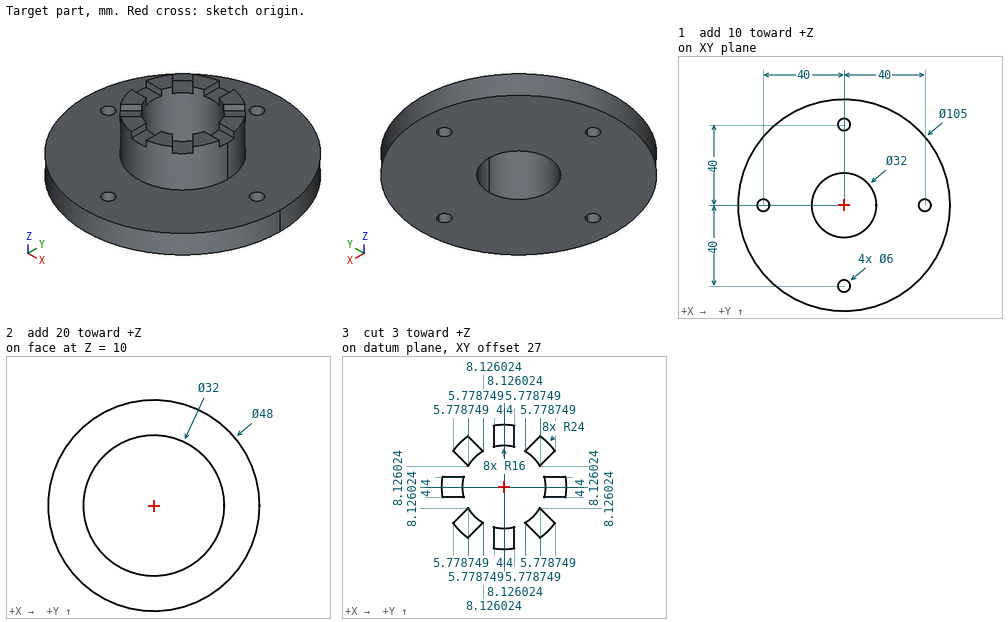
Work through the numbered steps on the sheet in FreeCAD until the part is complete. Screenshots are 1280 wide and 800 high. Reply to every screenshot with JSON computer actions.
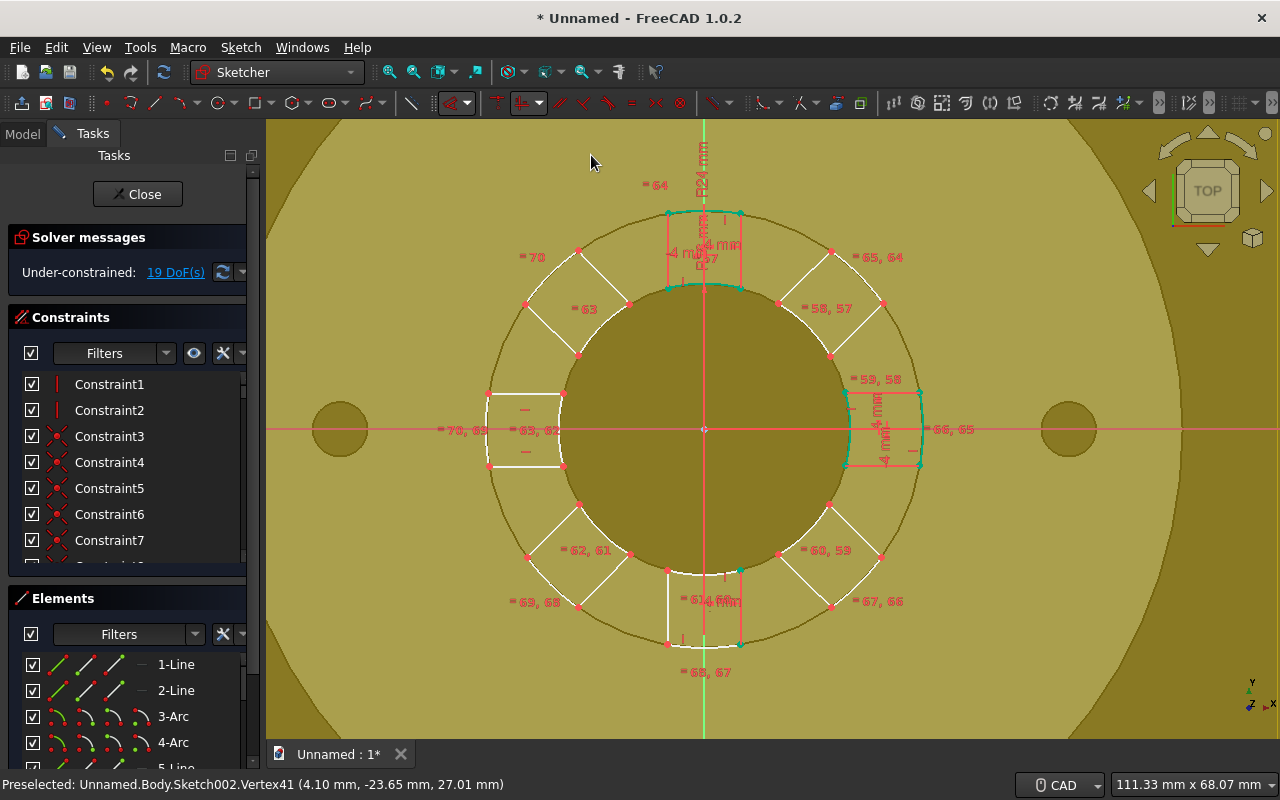
{"action": "left_click", "coordinate": [668, 570]}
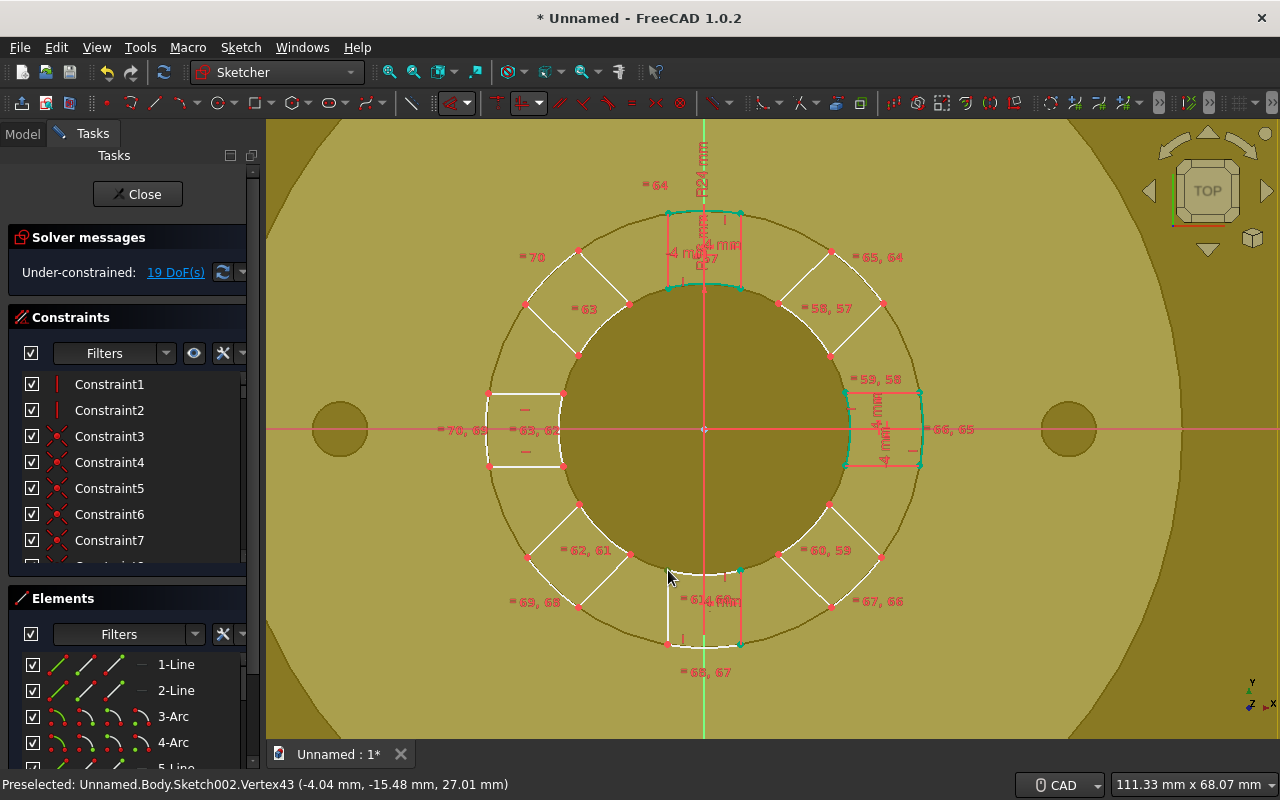
{"action": "left_click", "coordinate": [470, 104]}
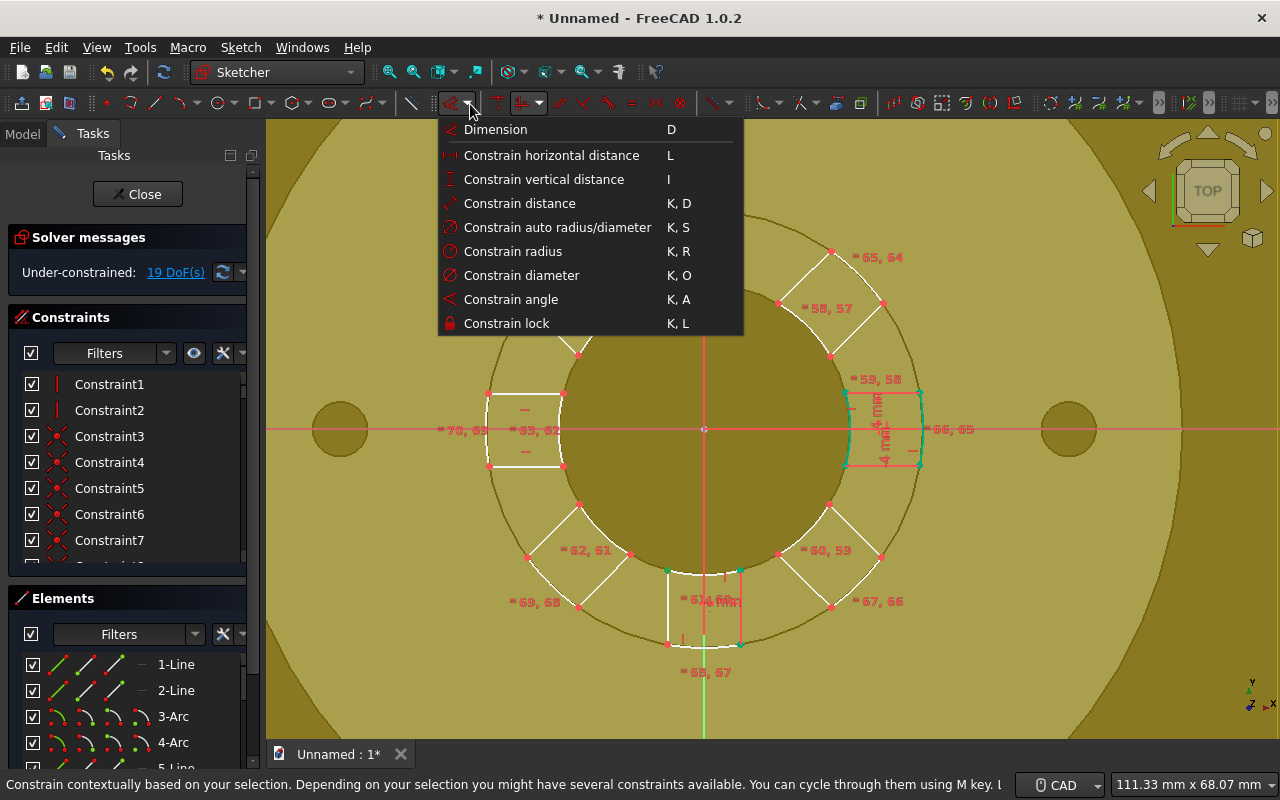
{"action": "left_click", "coordinate": [591, 155]}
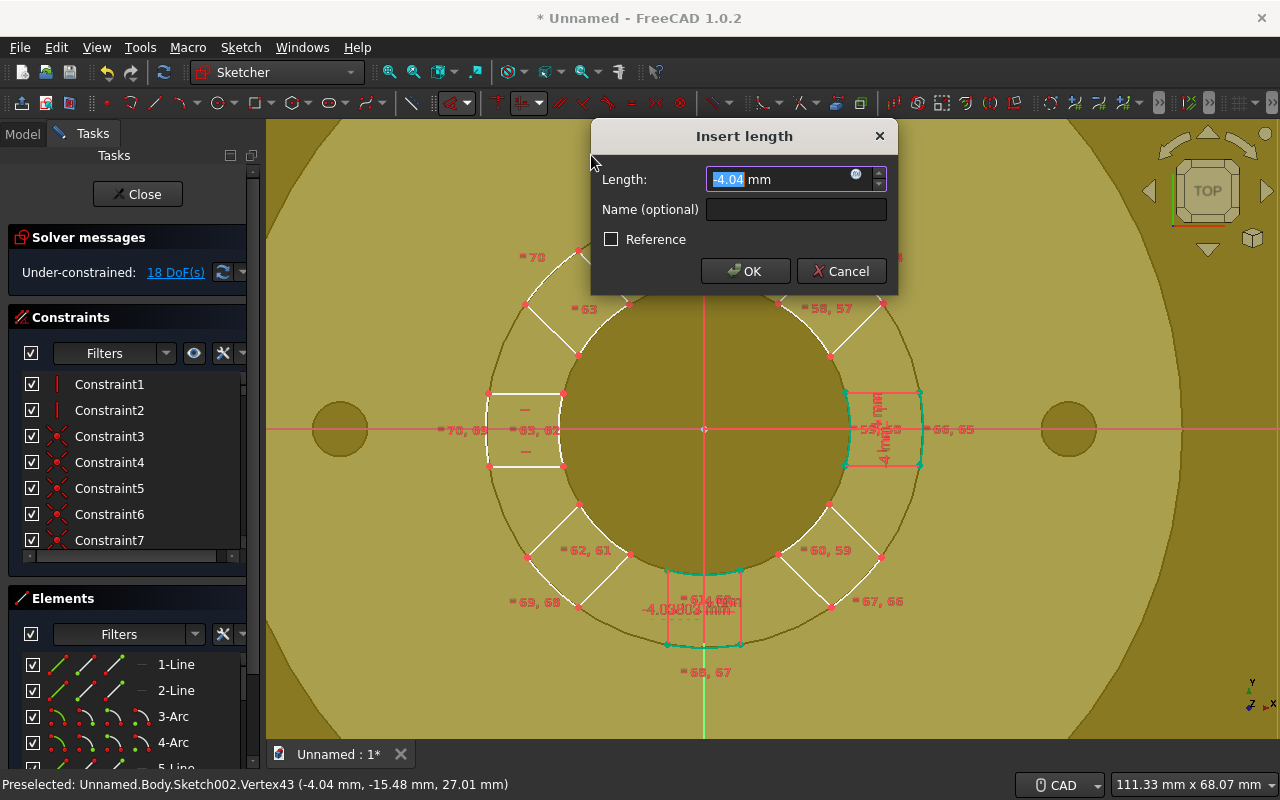
{"action": "type", "text": "-4"}
{"action": "key", "text": "Return"}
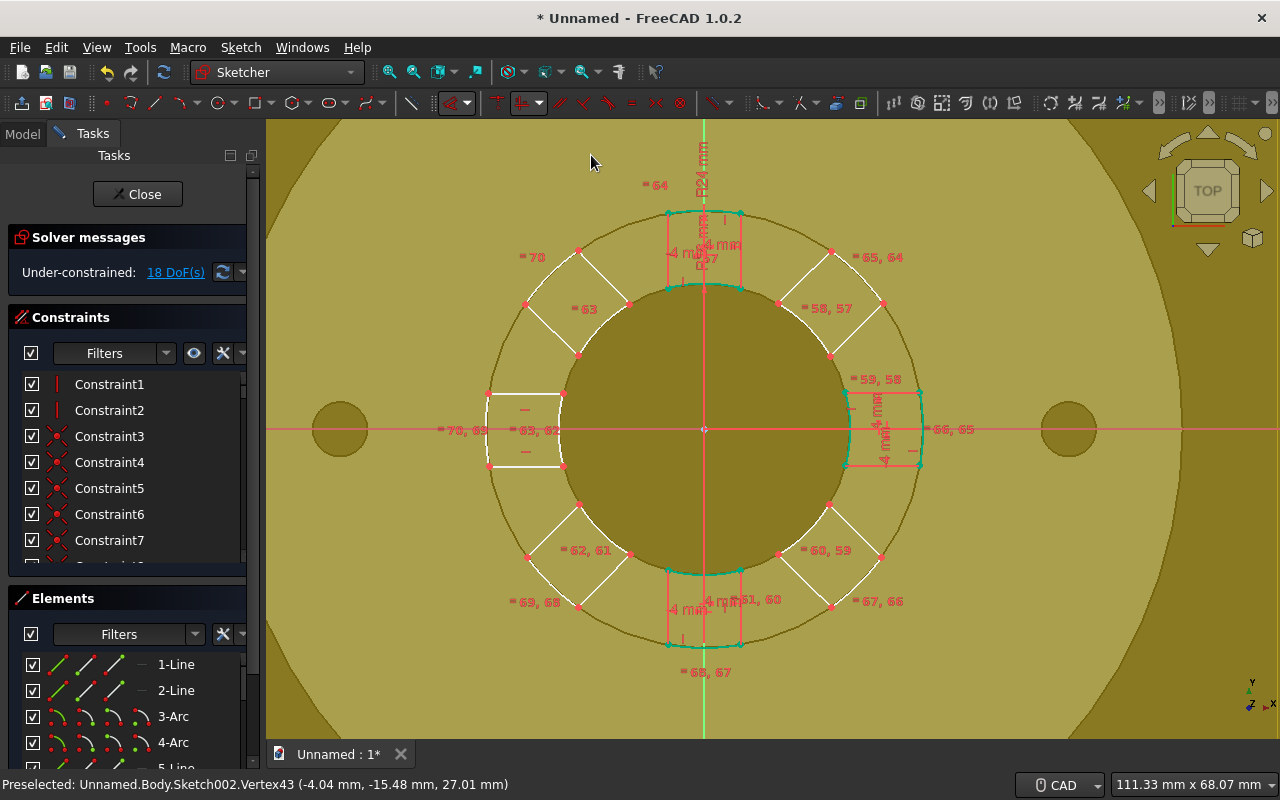
{"action": "left_click", "coordinate": [489, 467]}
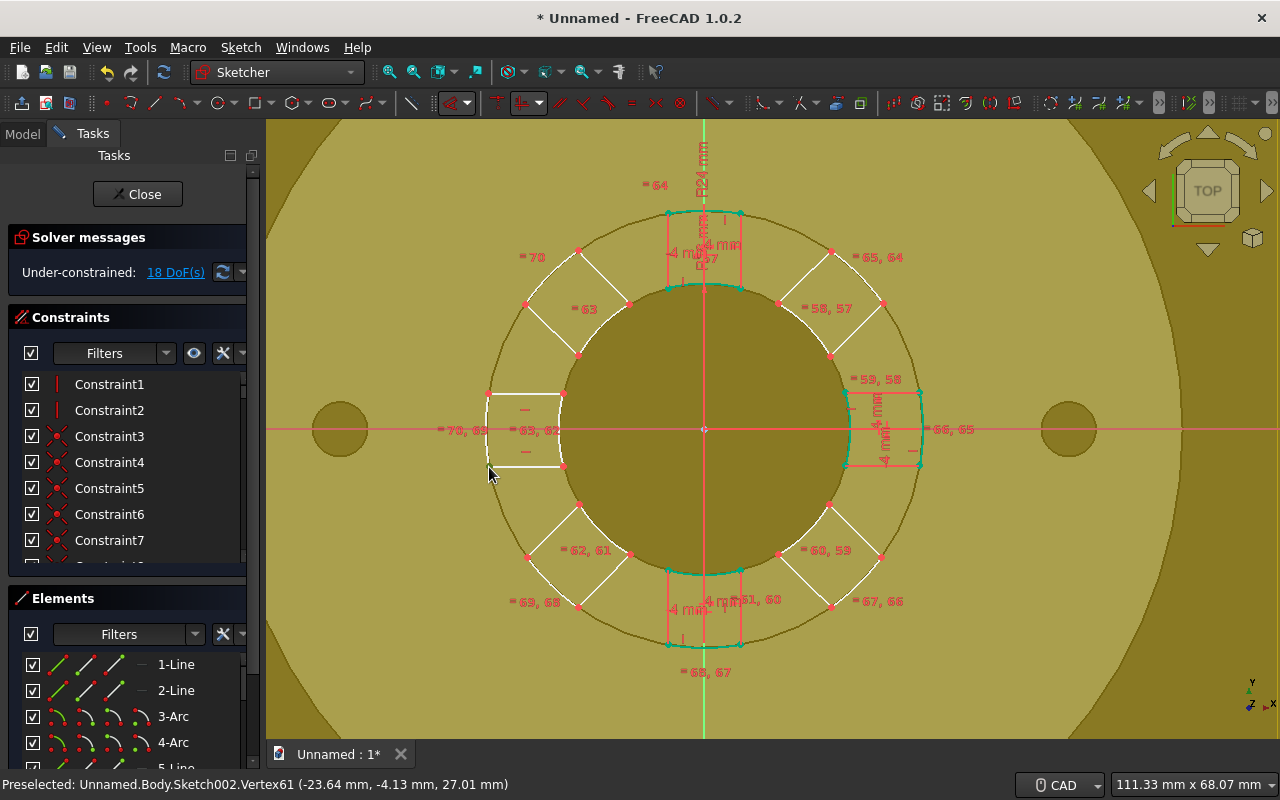
{"action": "left_click", "coordinate": [470, 104]}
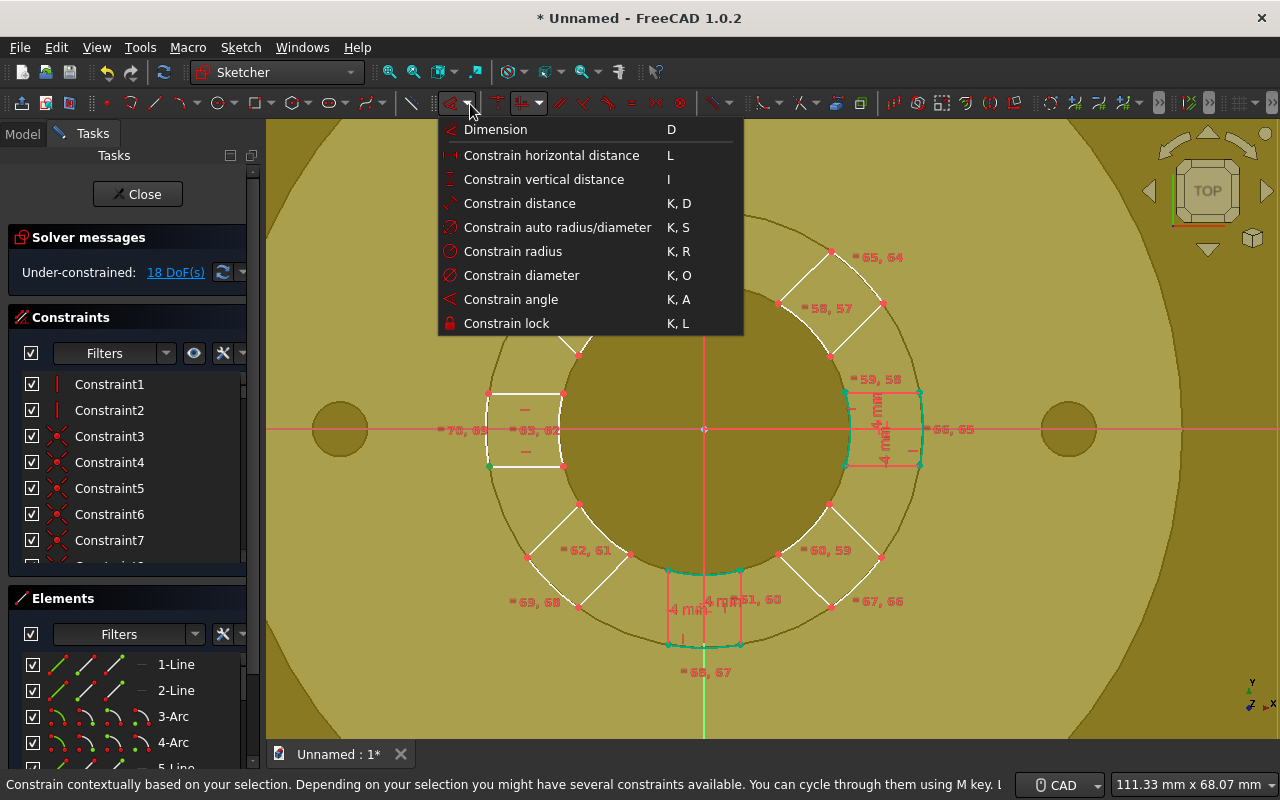
{"action": "left_click", "coordinate": [591, 179]}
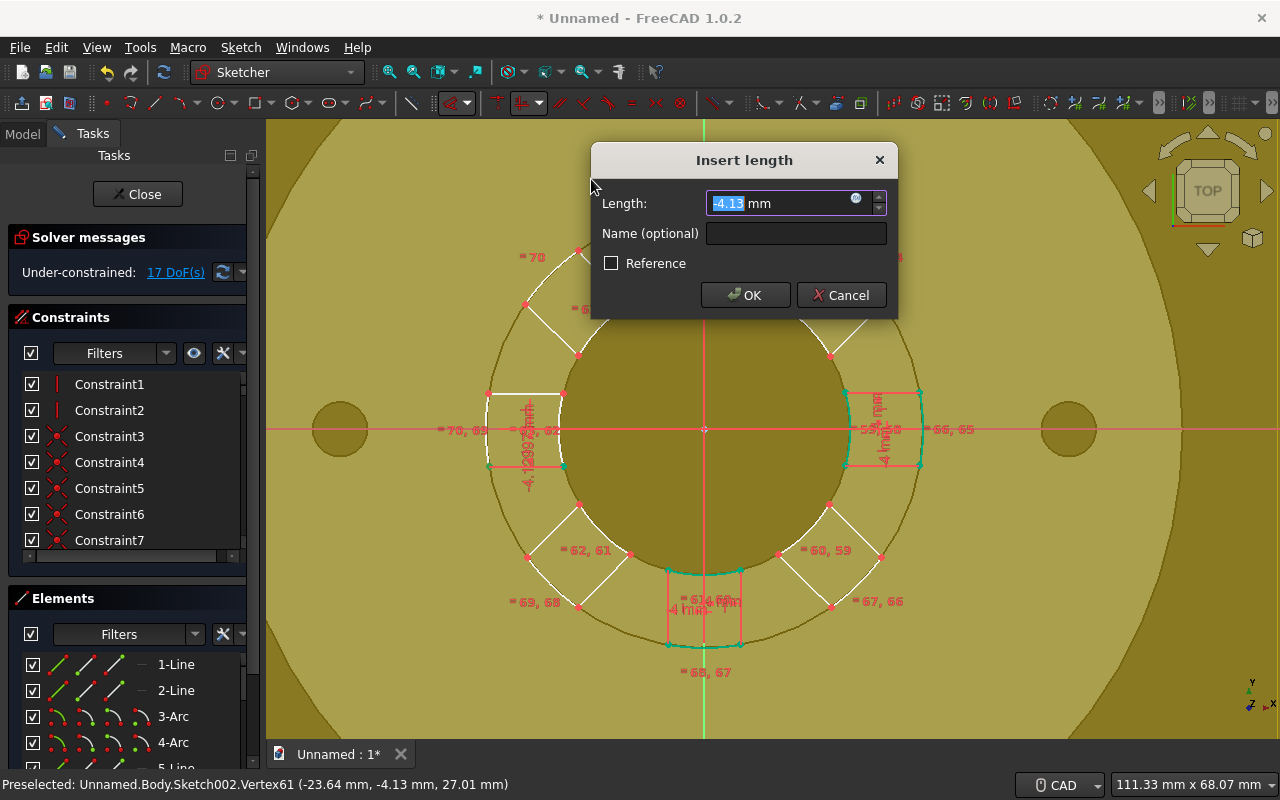
{"action": "type", "text": "-4"}
{"action": "key", "text": "Return"}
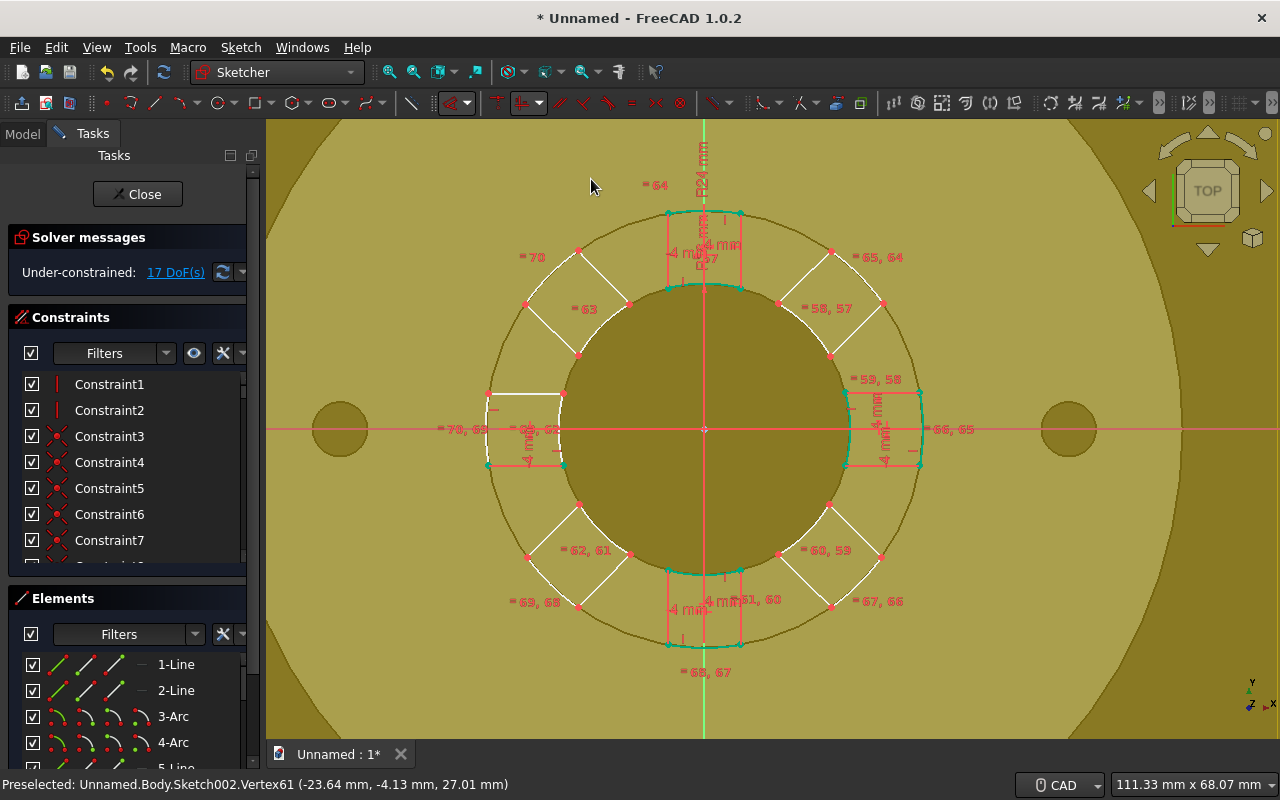
{"action": "left_click", "coordinate": [563, 394]}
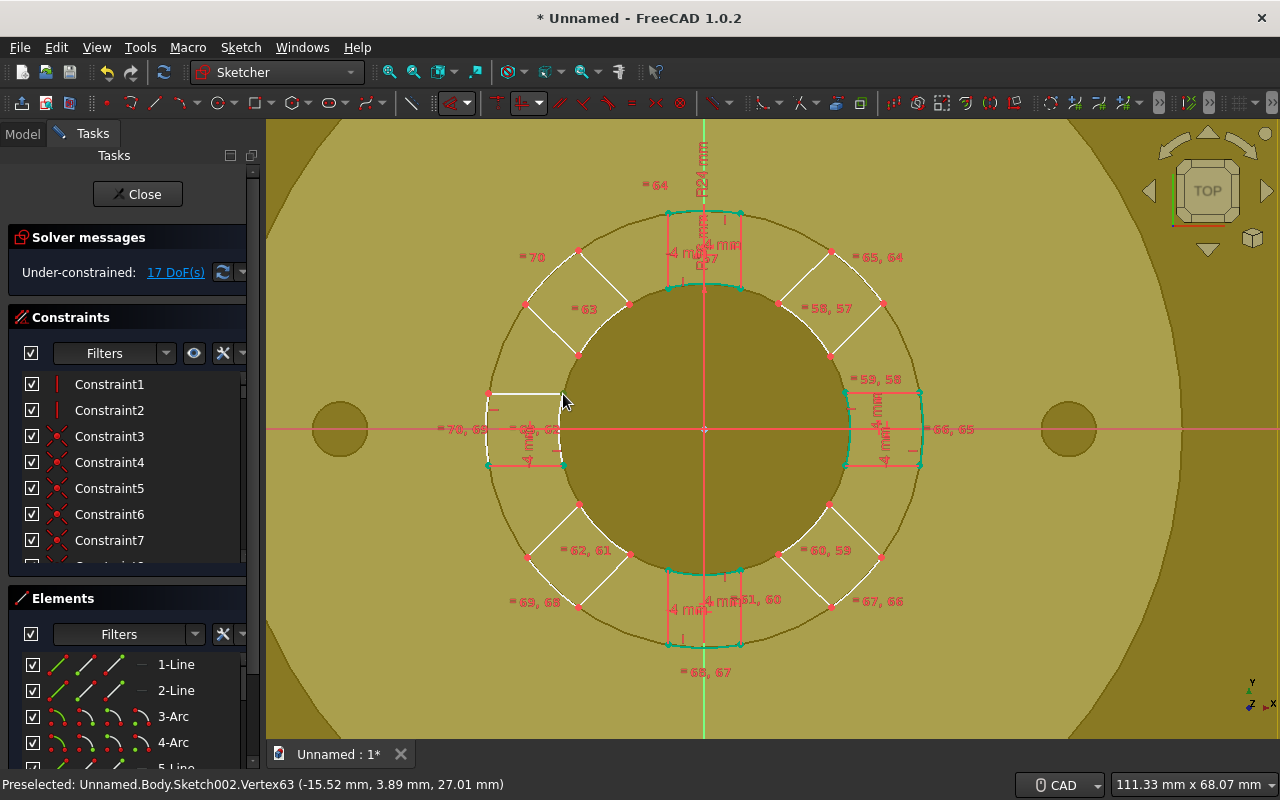
{"action": "left_click", "coordinate": [470, 104]}